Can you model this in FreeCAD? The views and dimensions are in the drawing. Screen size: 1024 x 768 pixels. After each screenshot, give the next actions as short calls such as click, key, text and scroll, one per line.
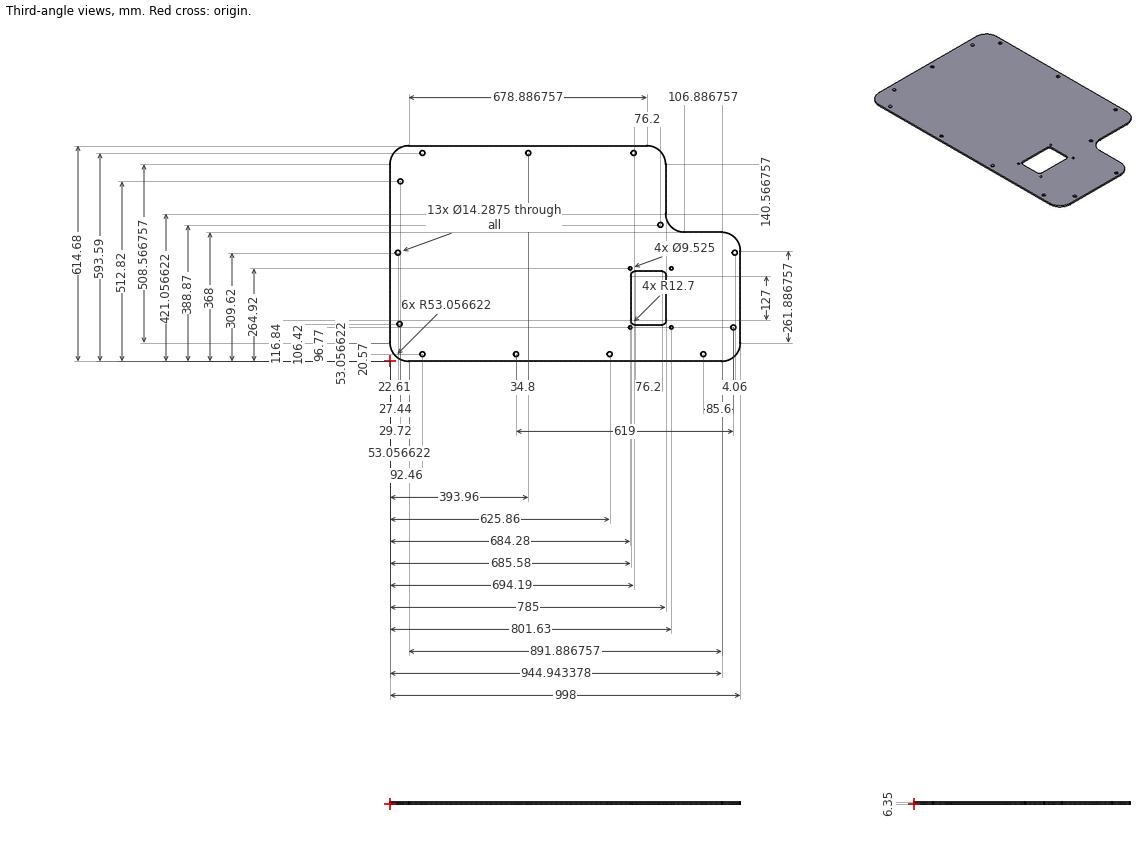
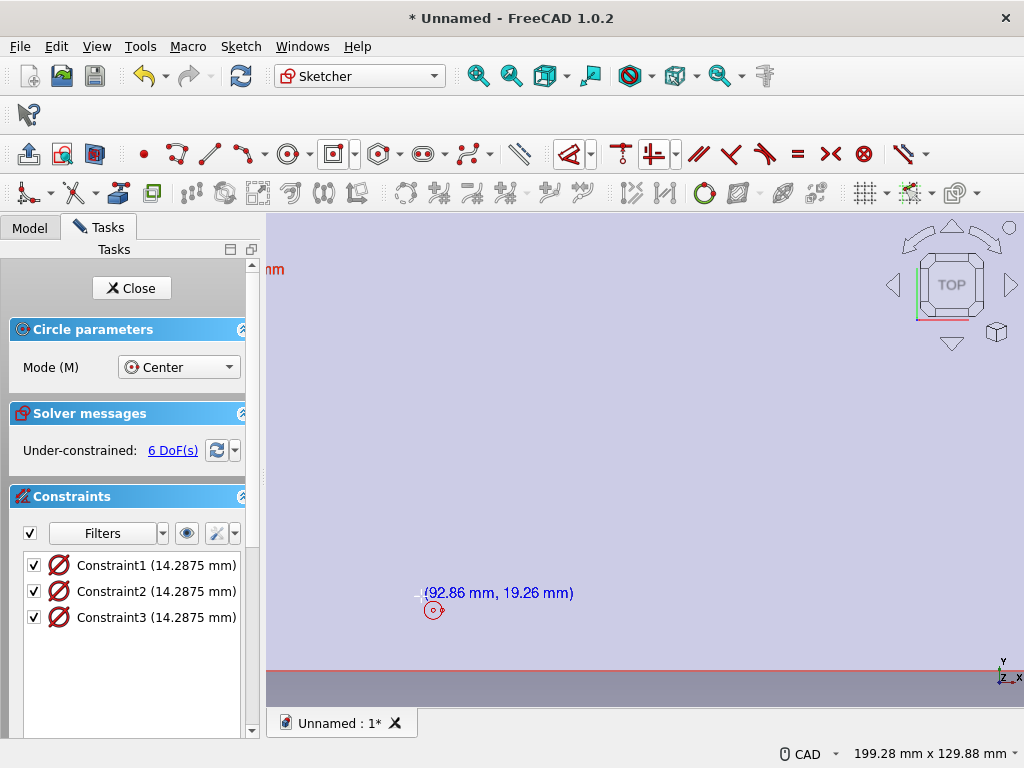
scroll(406, 576, down, 11)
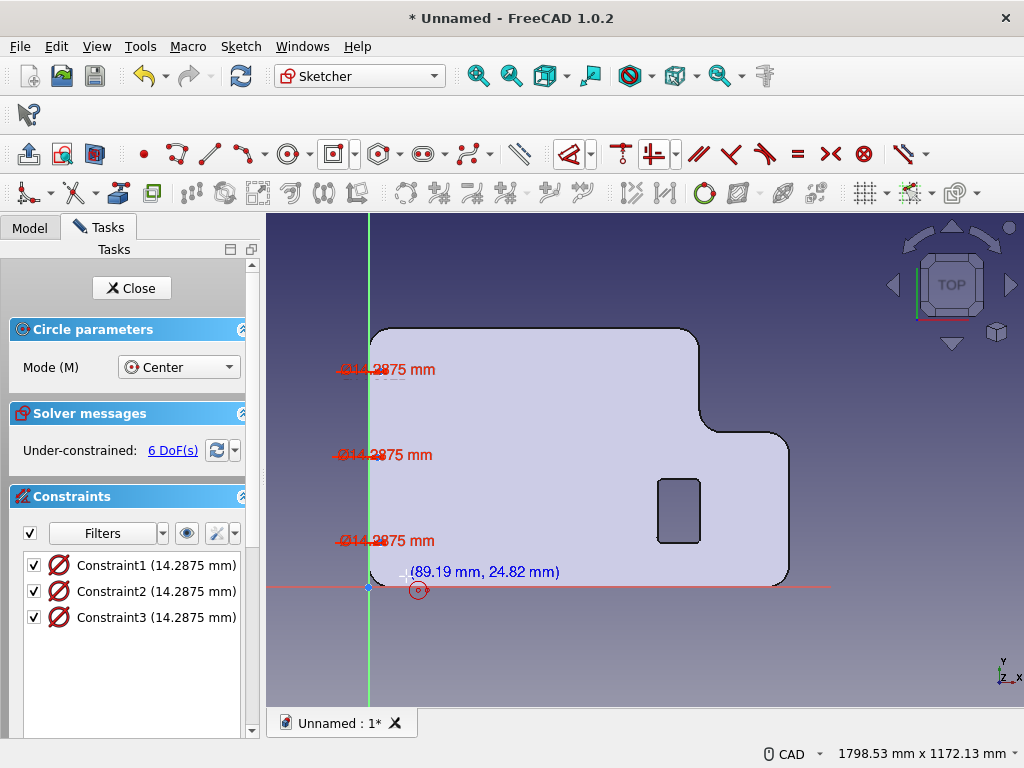
scroll(408, 579, up, 4)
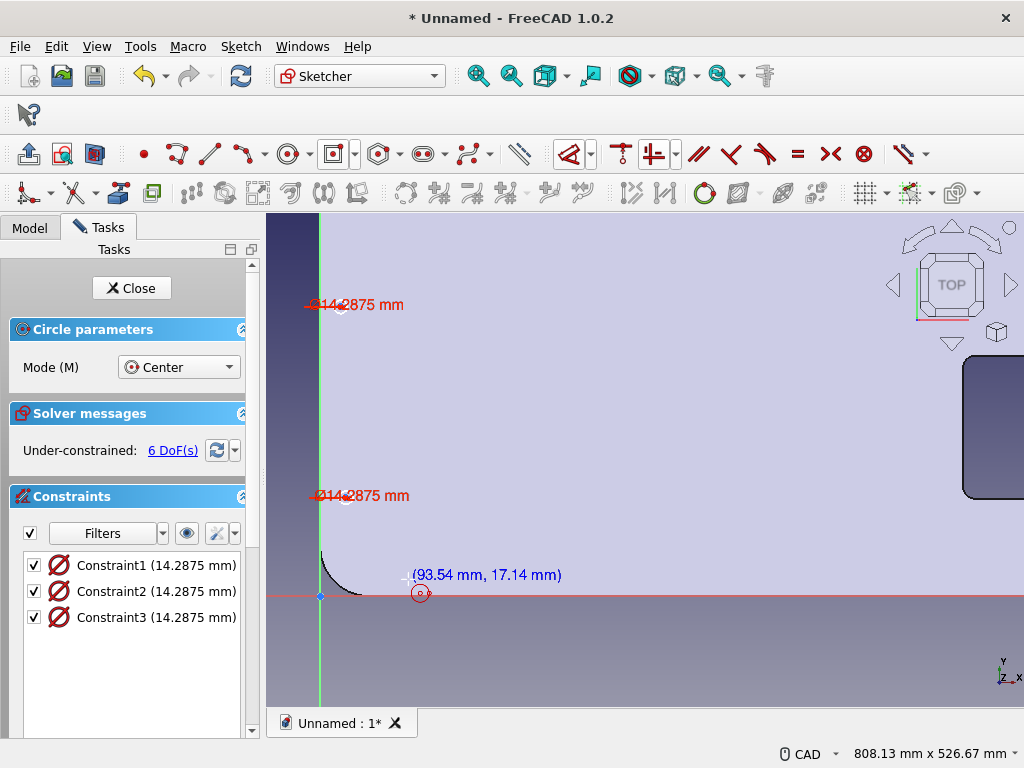
click(407, 577)
move(411, 572)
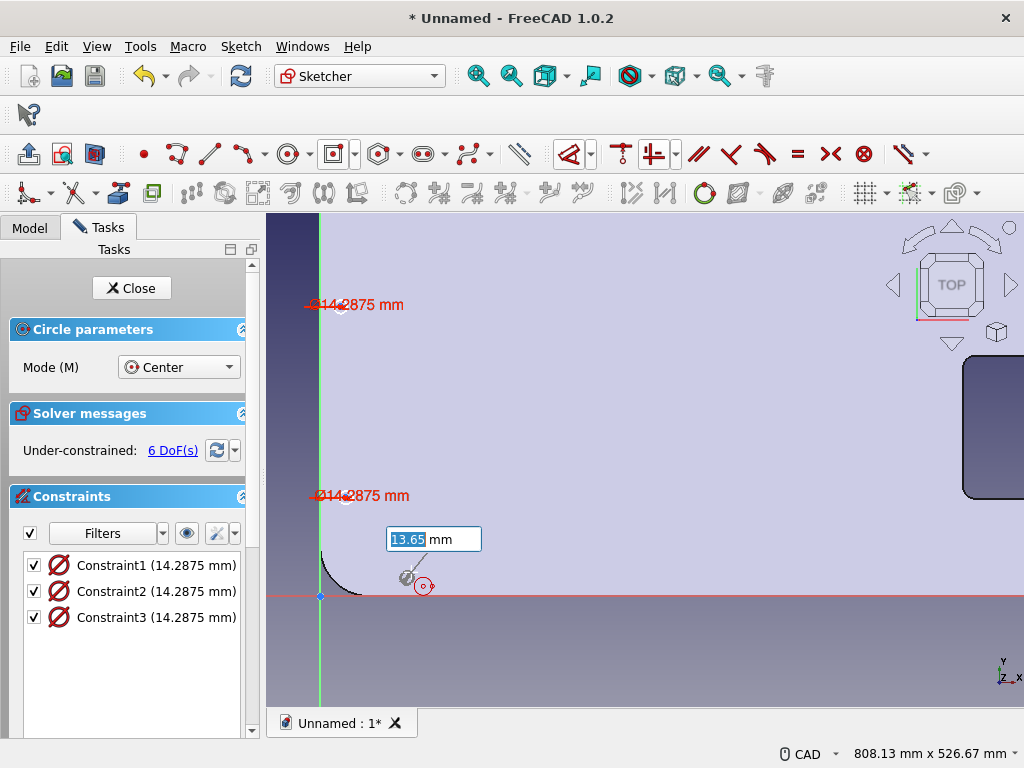
text(14.2875)
key(Return)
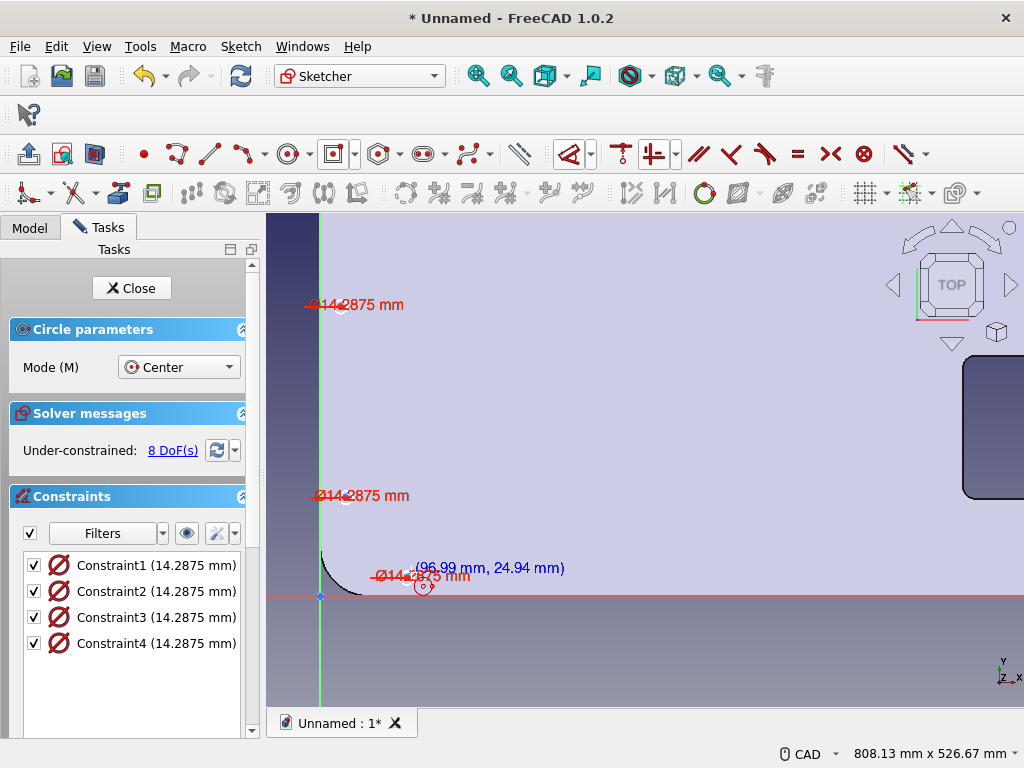
scroll(407, 579, down, 4)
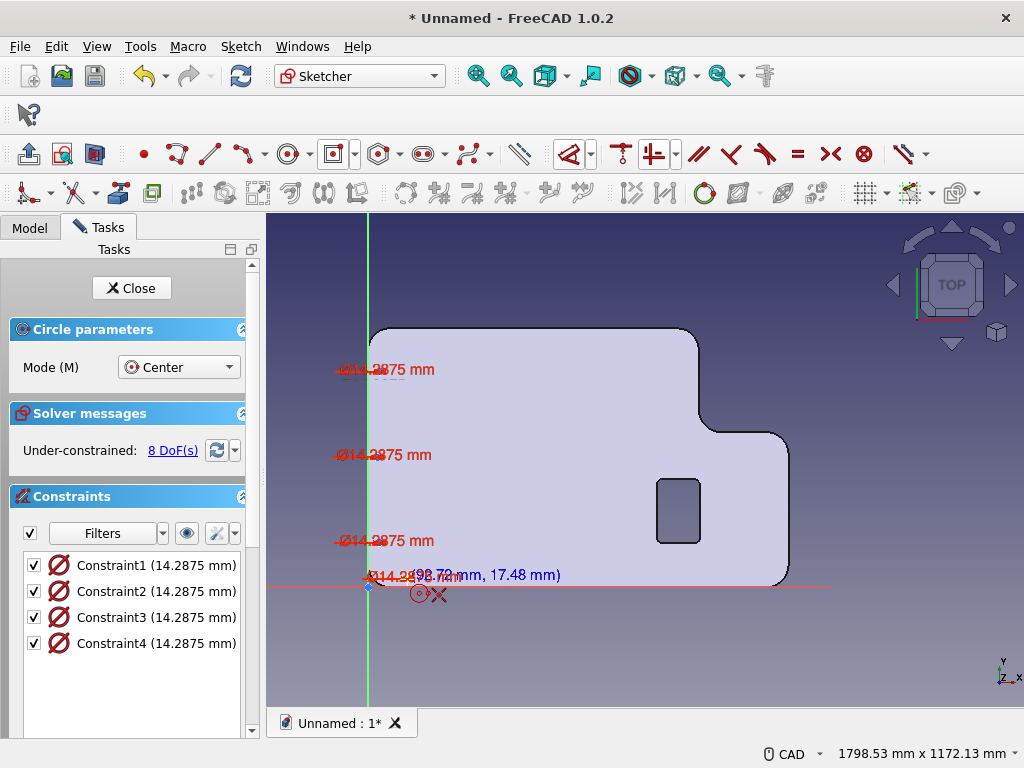
scroll(407, 337, up, 11)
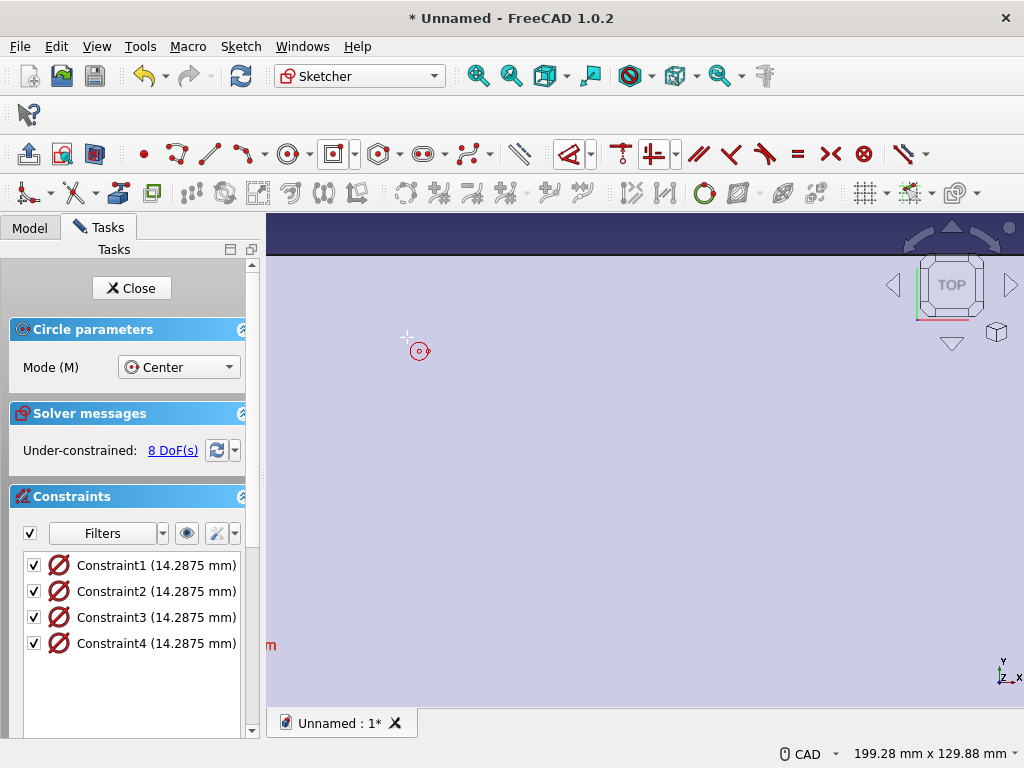
scroll(407, 337, down, 11)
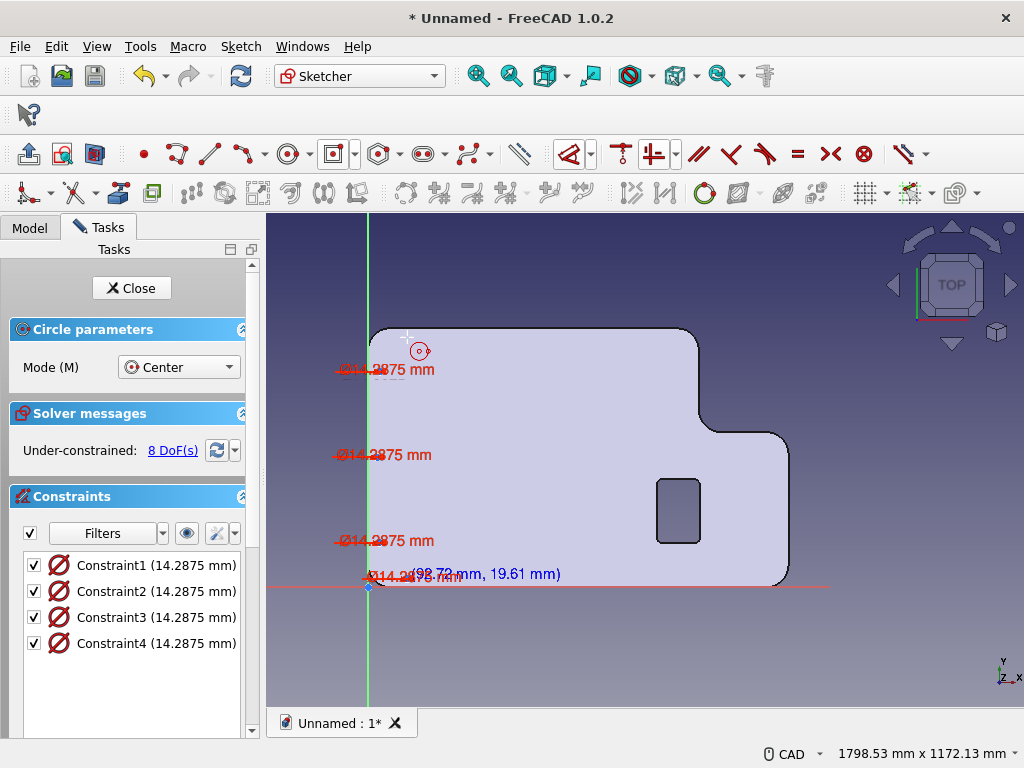
click(407, 337)
move(409, 335)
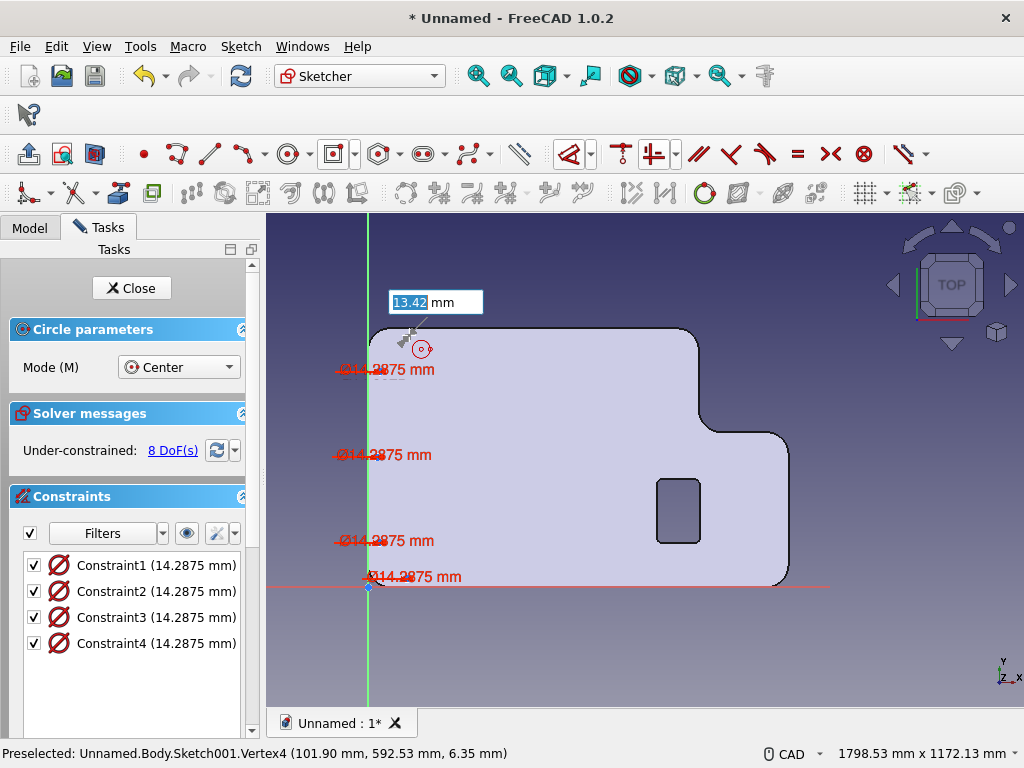
text(14.2875)
key(Return)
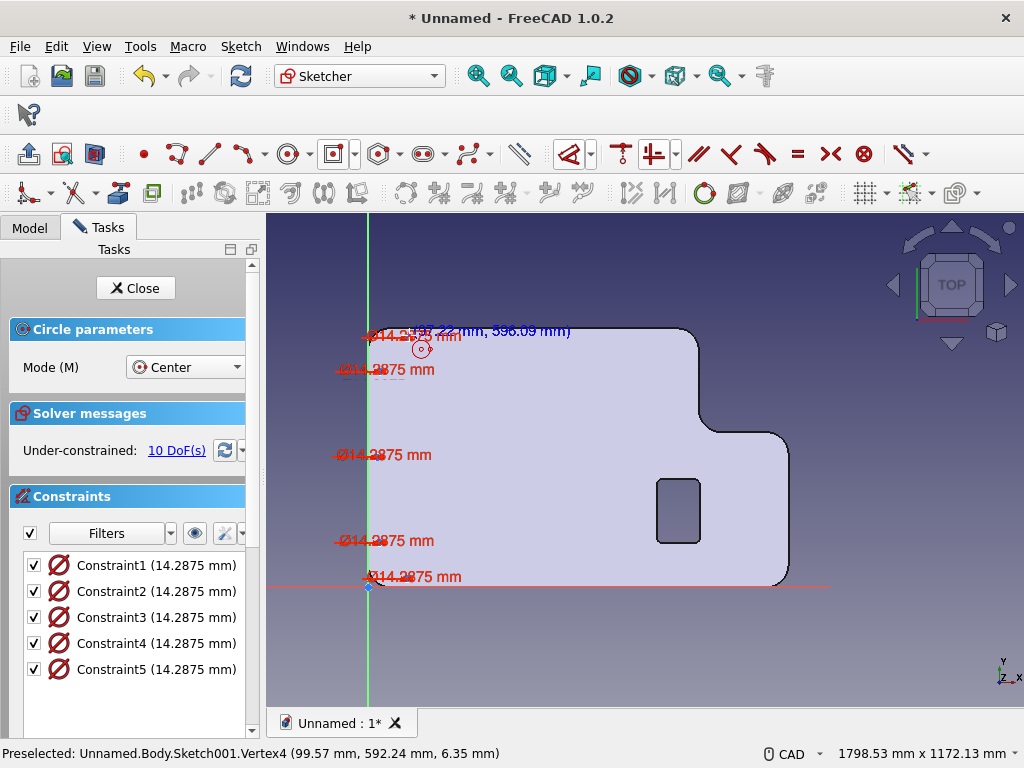
scroll(661, 337, up, 11)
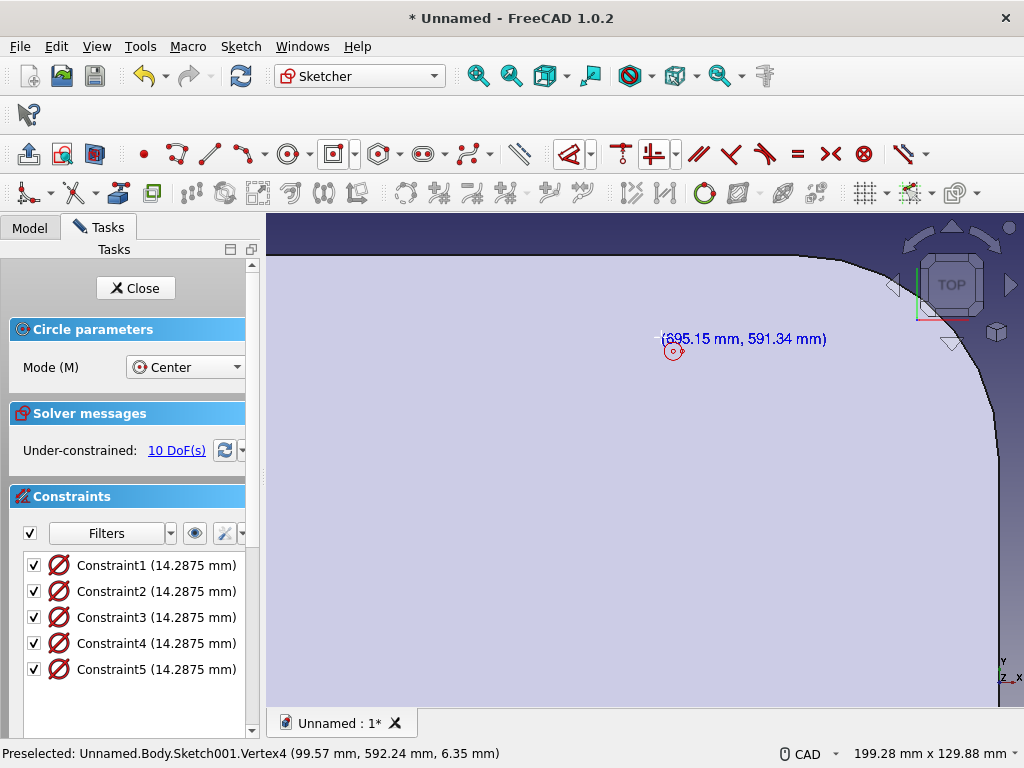
scroll(662, 337, down, 11)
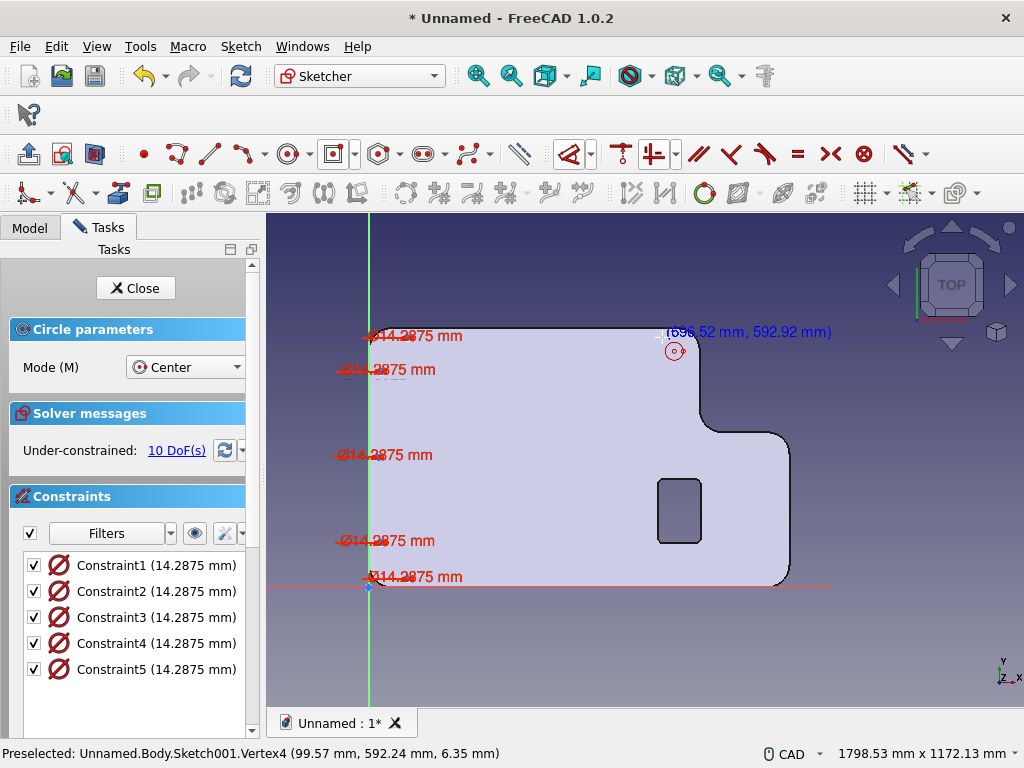
click(661, 337)
move(664, 335)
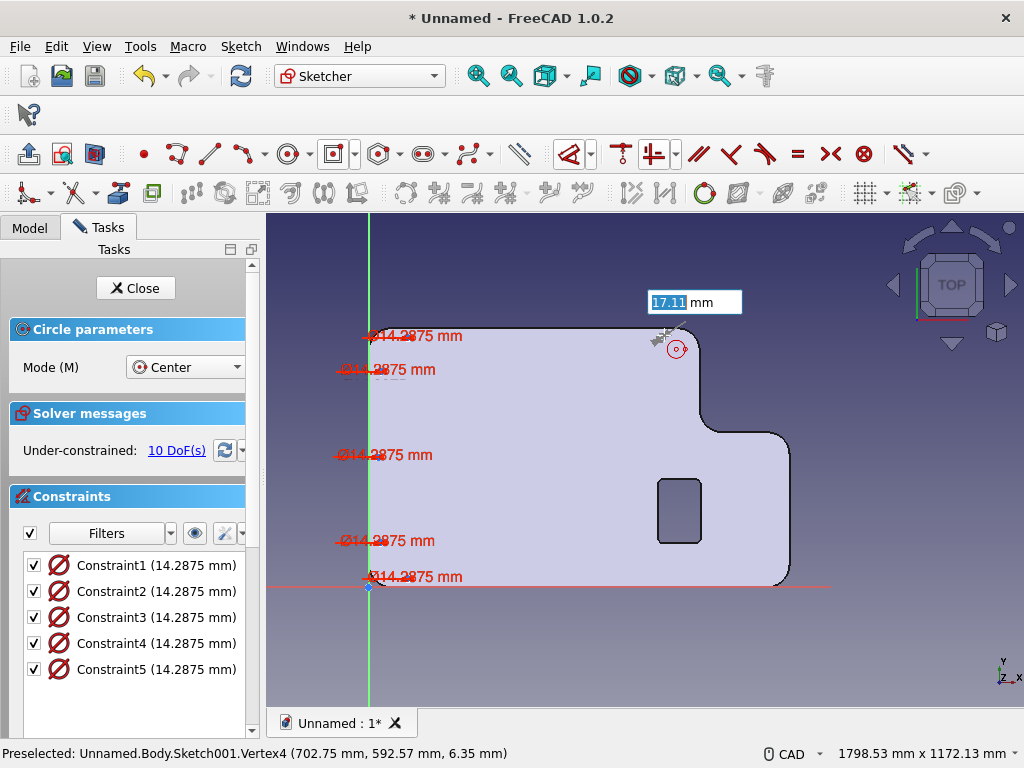
text(14.2875)
key(Return)